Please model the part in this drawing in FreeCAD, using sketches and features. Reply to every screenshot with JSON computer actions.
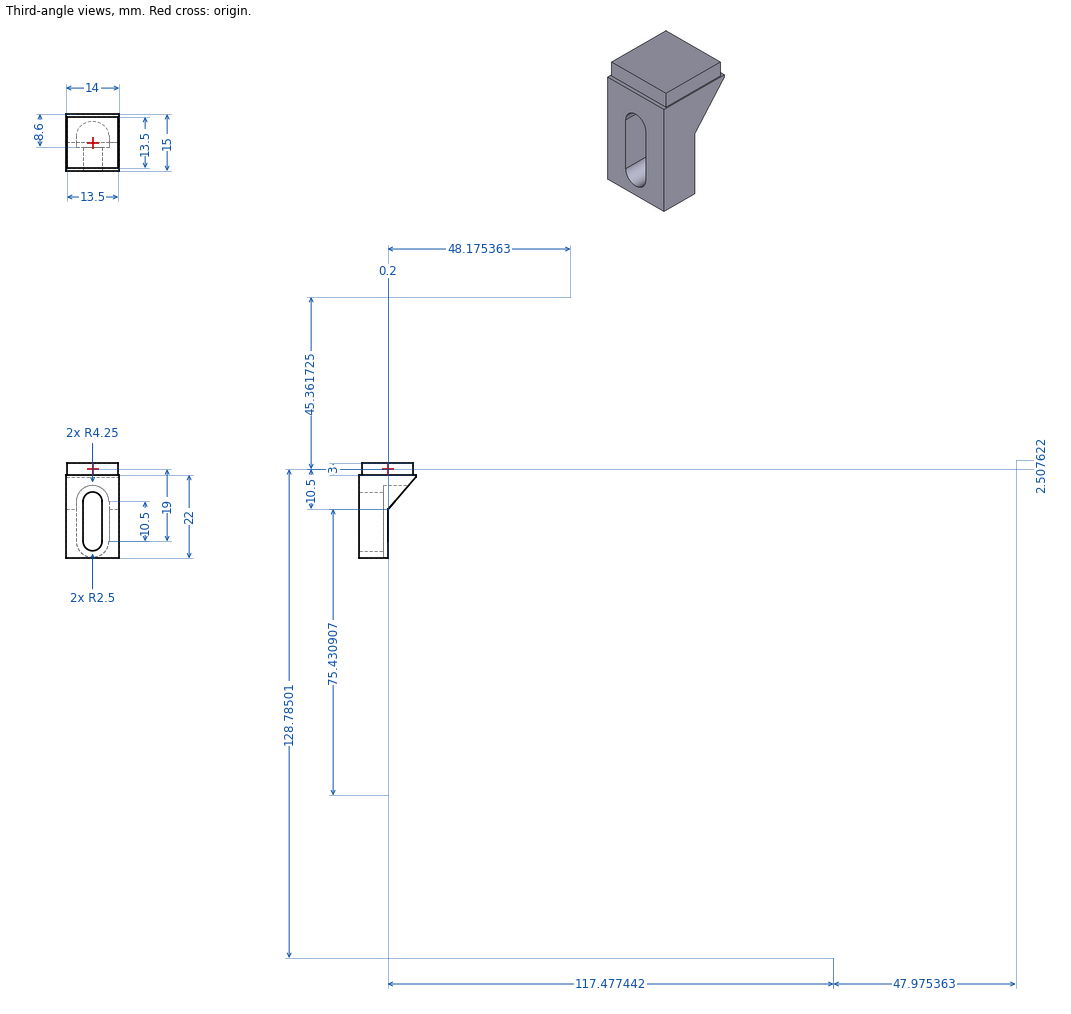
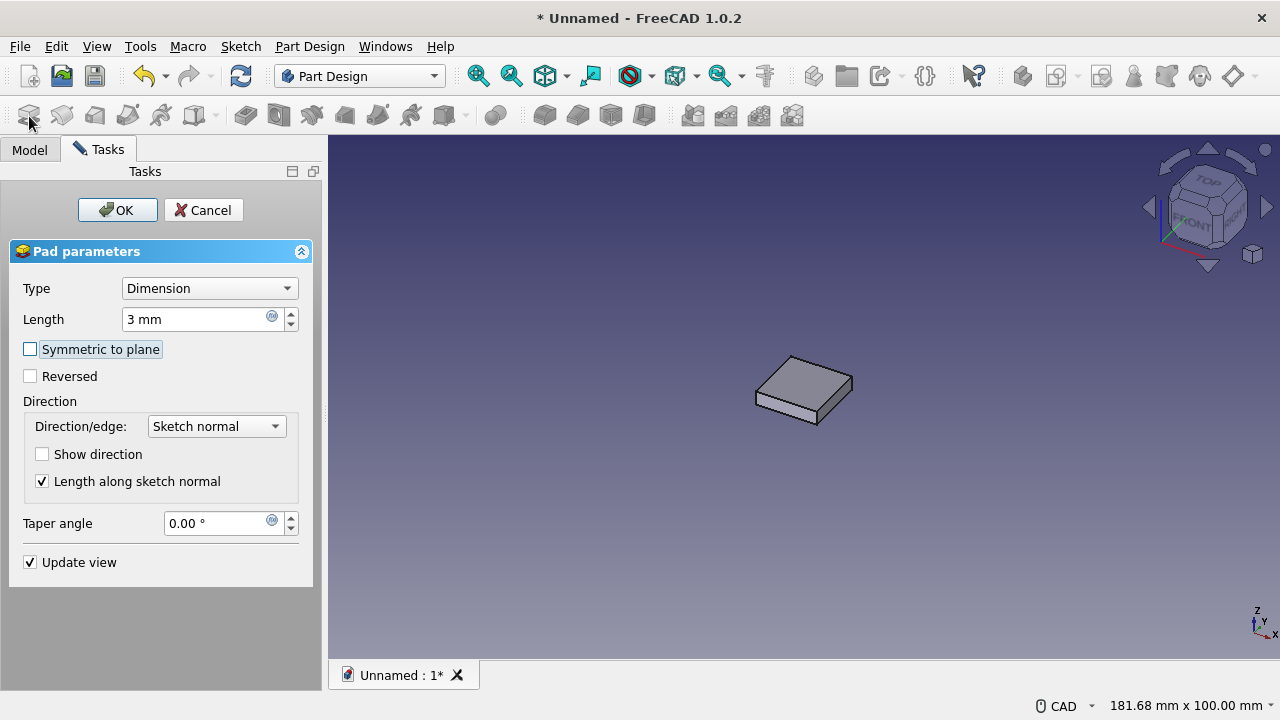
{"action": "left_click", "coordinate": [31, 349]}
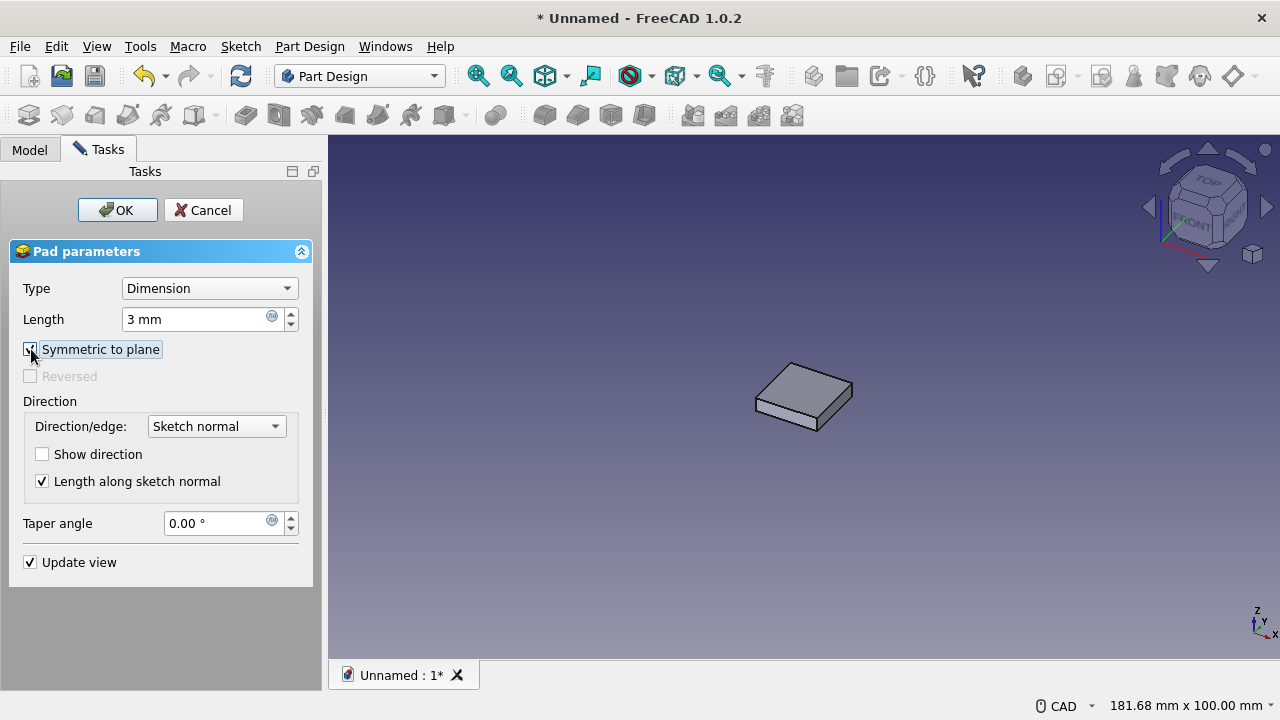
{"action": "left_click", "coordinate": [118, 210]}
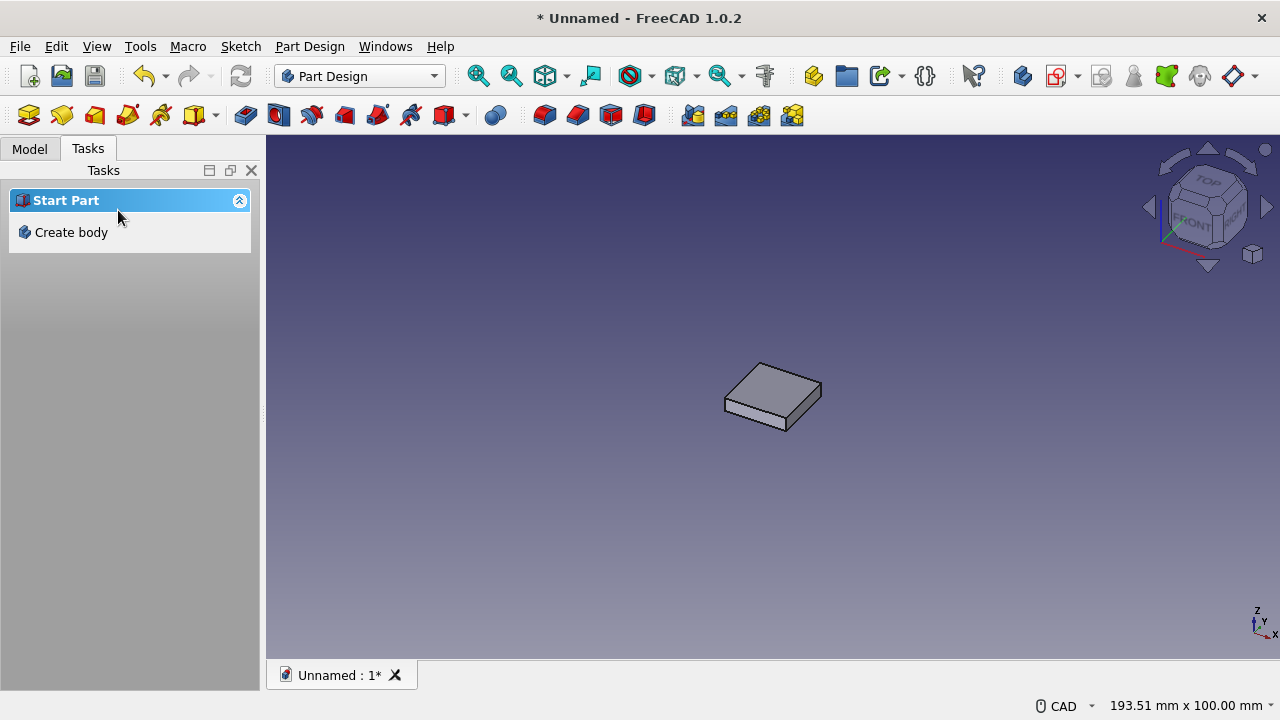
{"action": "left_click", "coordinate": [479, 76]}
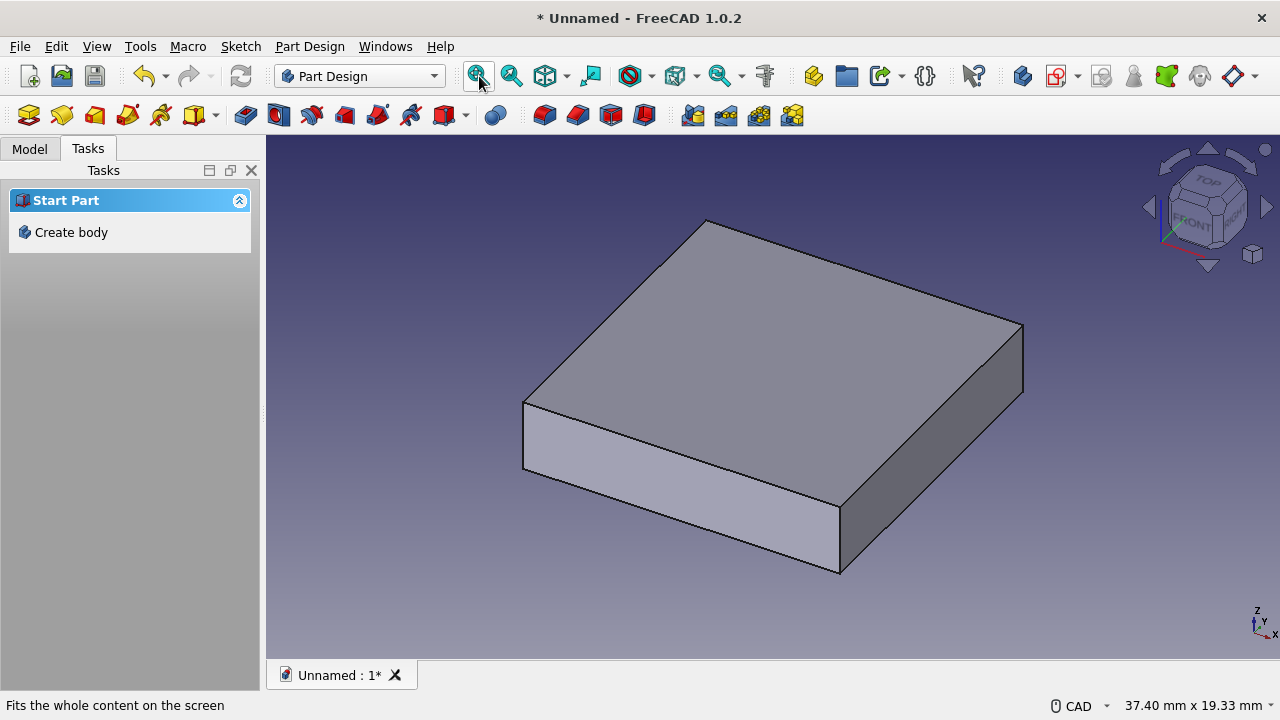
{"action": "key", "text": "5"}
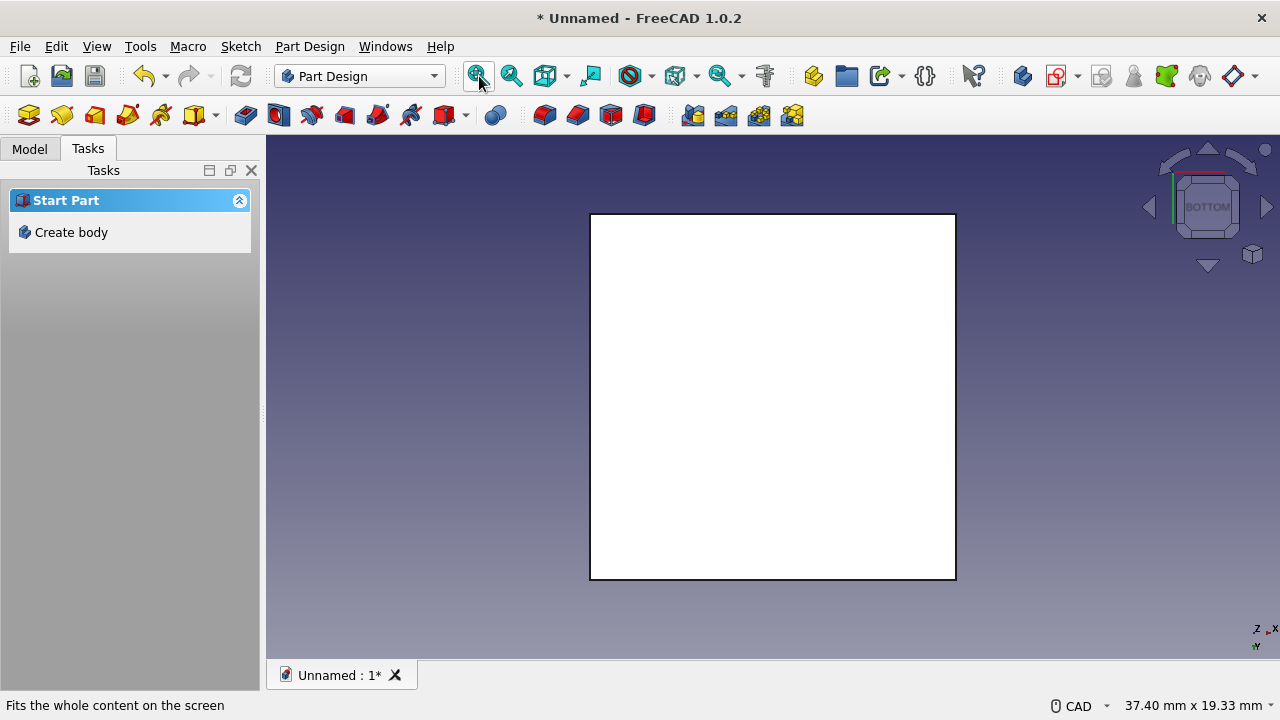
{"action": "left_click", "coordinate": [773, 396]}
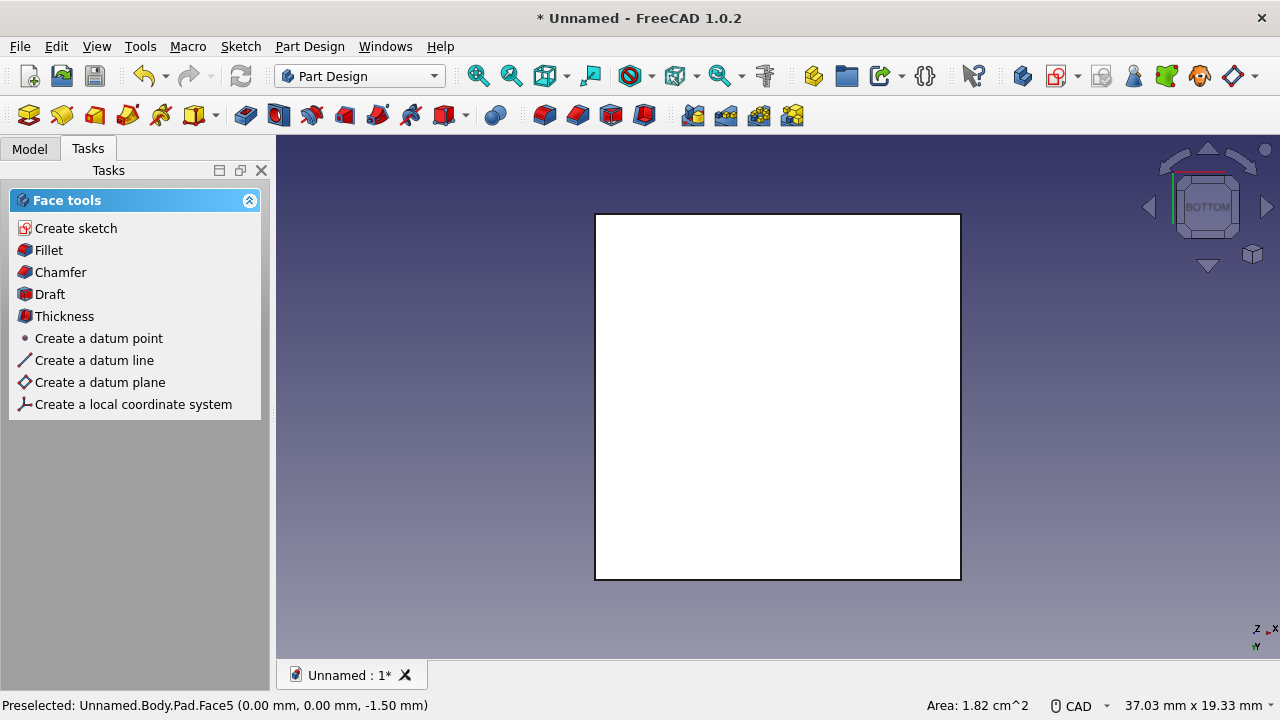
{"action": "left_click", "coordinate": [1056, 76]}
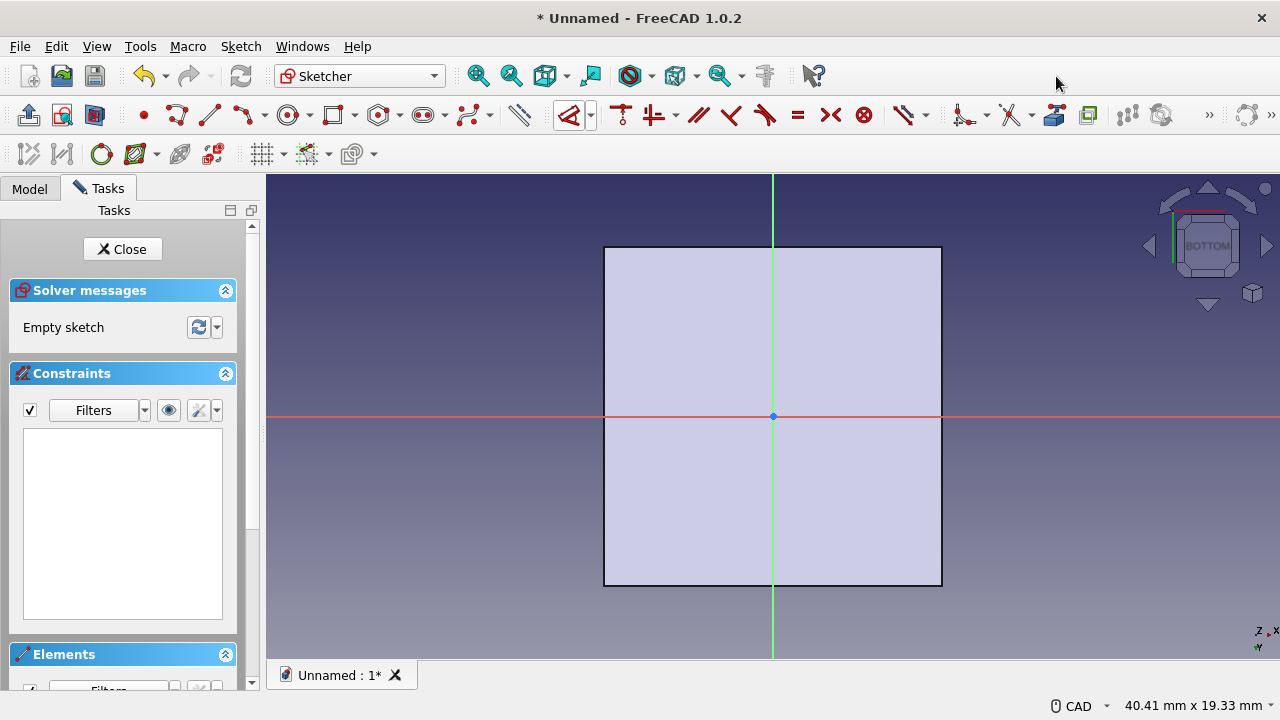
{"action": "key", "text": "g v"}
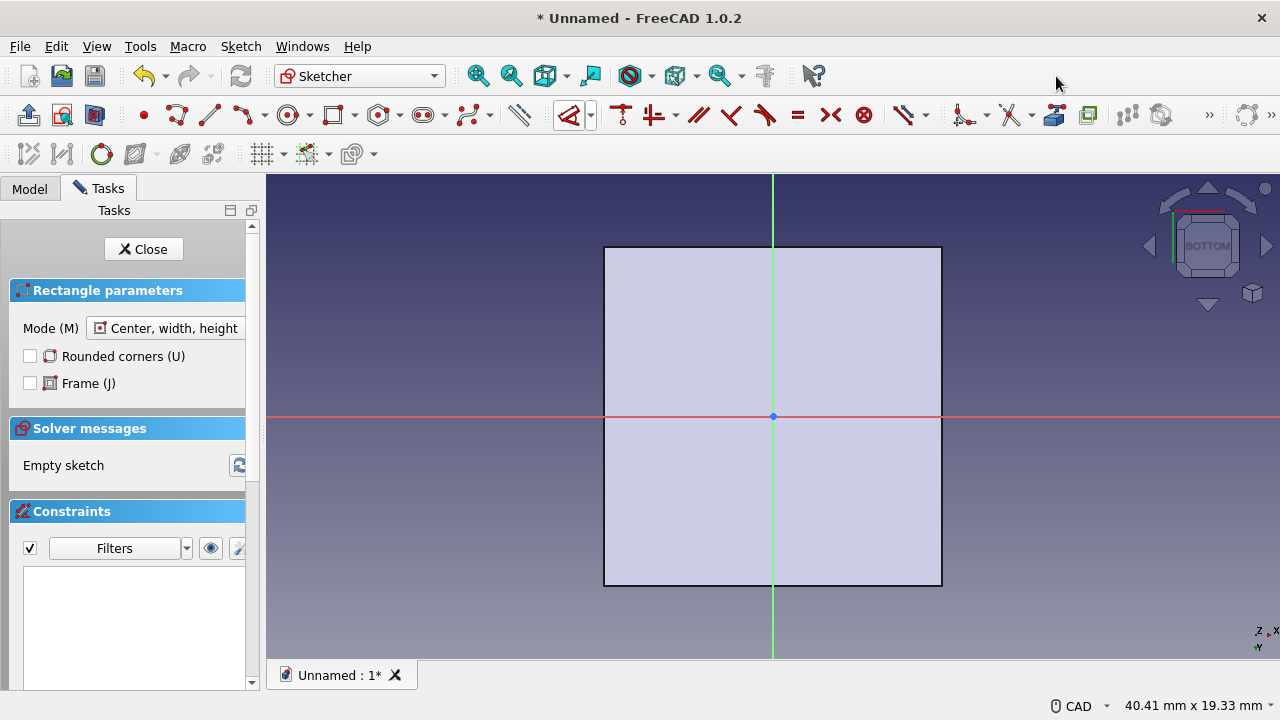
{"action": "left_click", "coordinate": [773, 416]}
{"action": "mouse_move", "coordinate": [949, 228]}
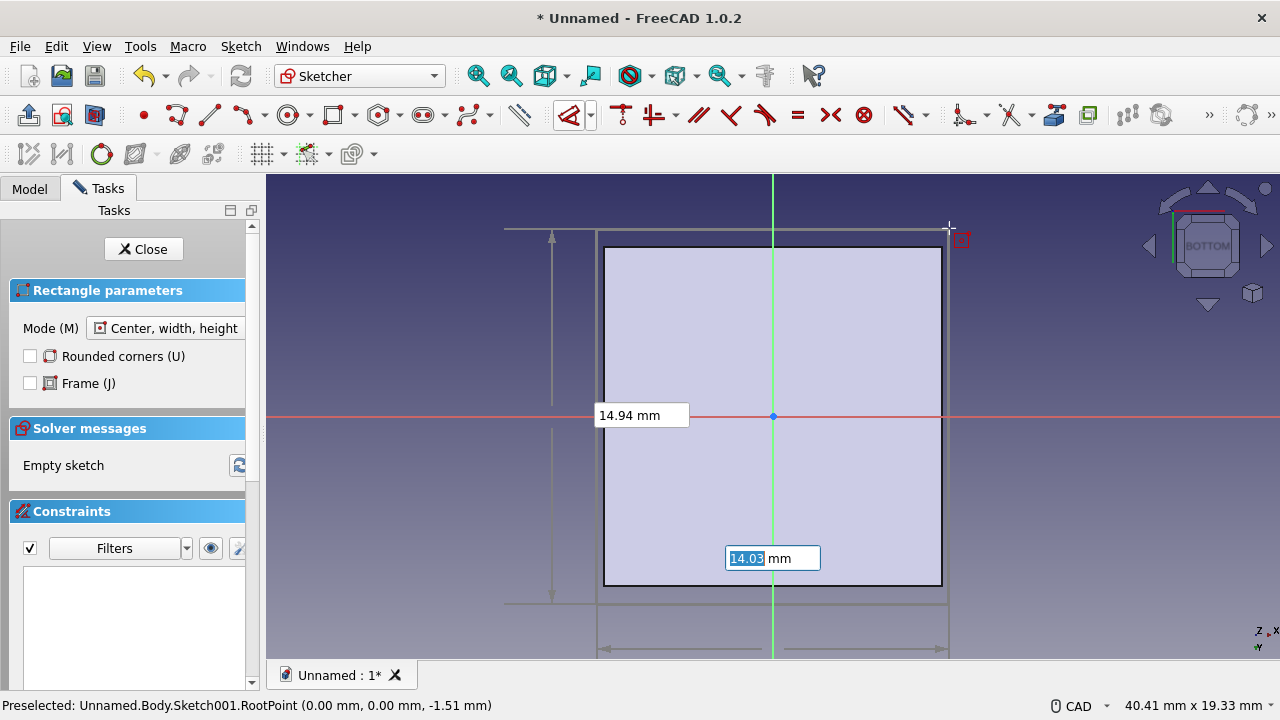
{"action": "type", "text": "14"}
{"action": "key", "text": "Tab"}
{"action": "type", "text": "15"}
{"action": "key", "text": "Return"}
{"action": "key", "text": "Escape"}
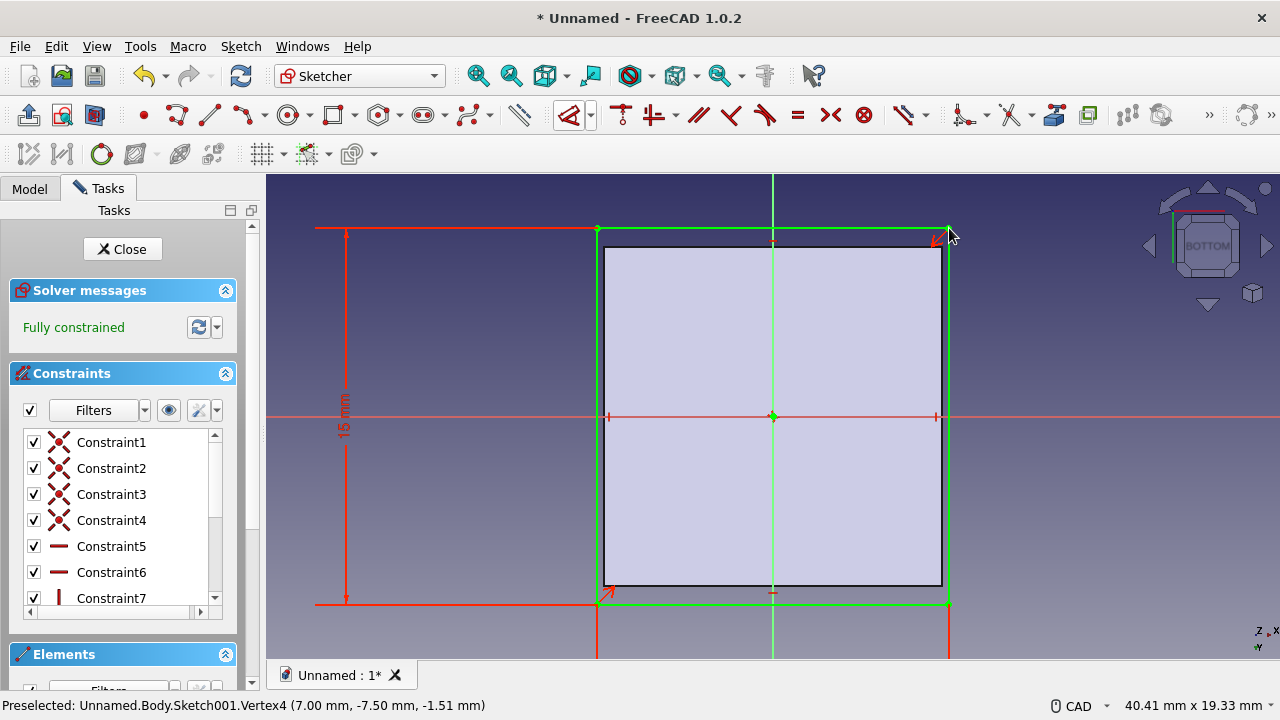
{"action": "left_click", "coordinate": [123, 249]}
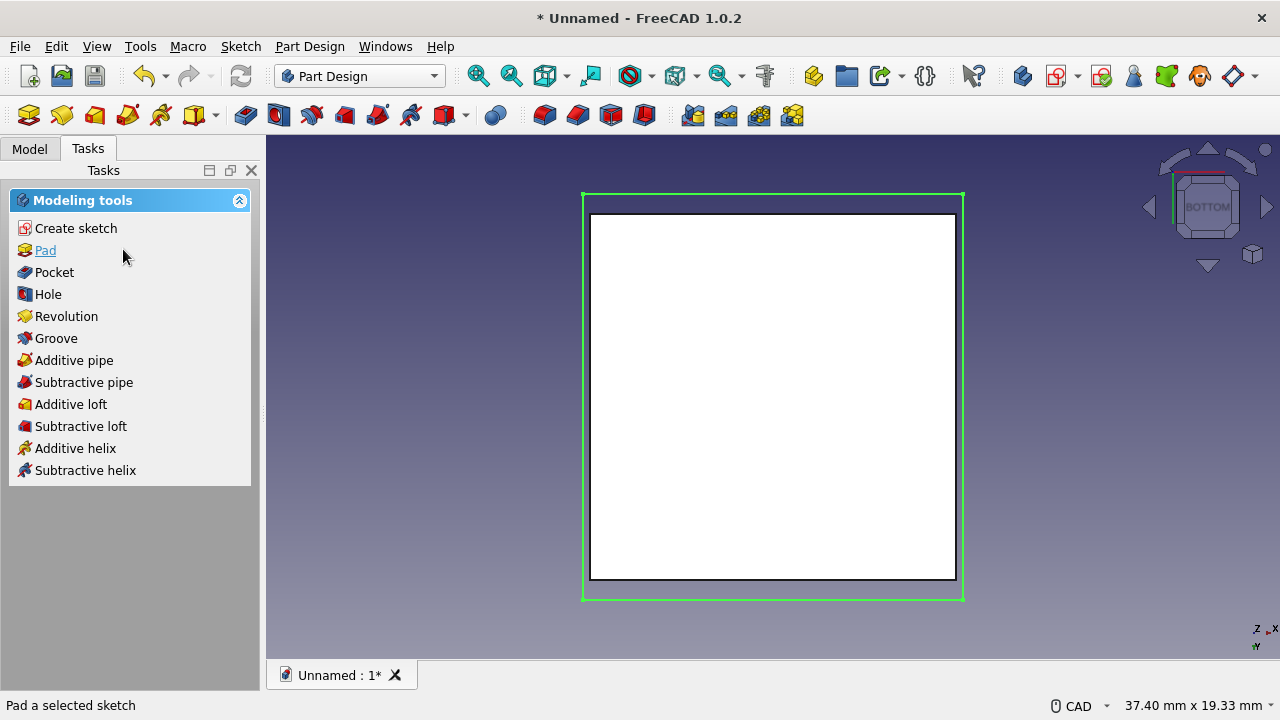
{"action": "left_click", "coordinate": [29, 116]}